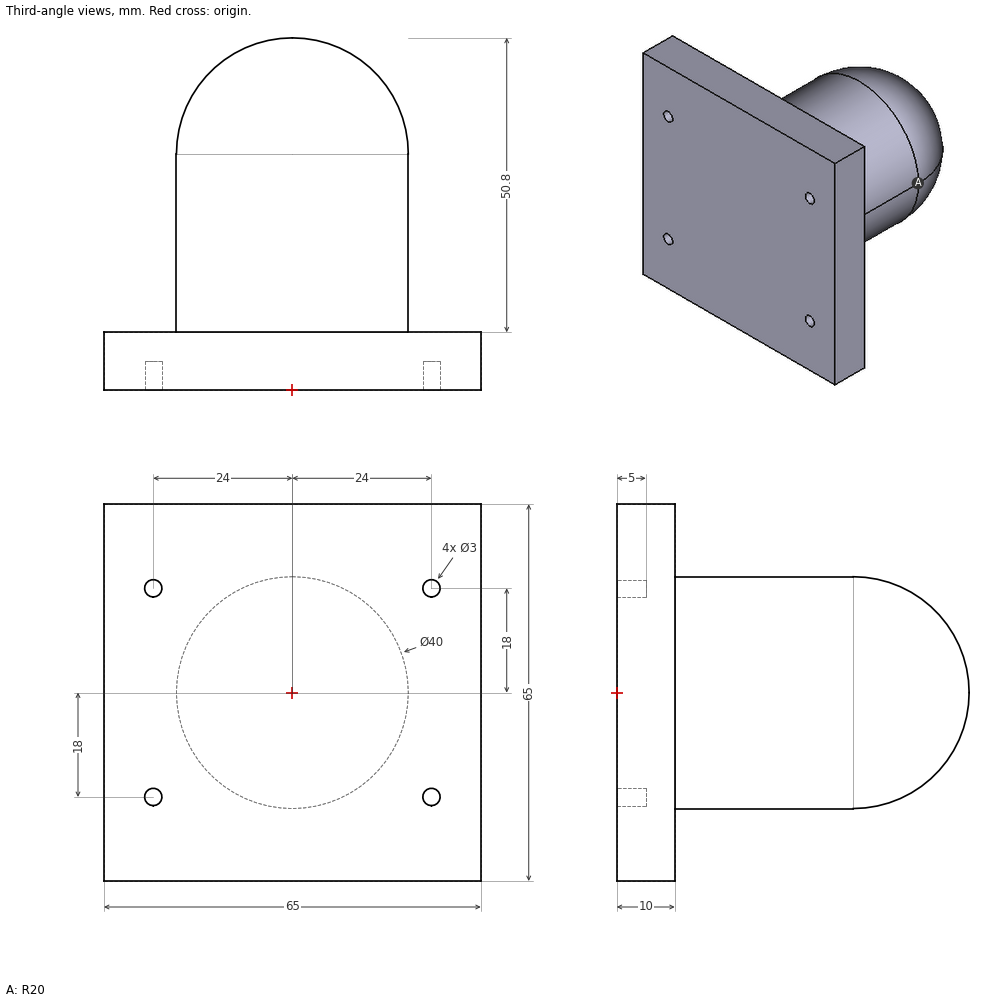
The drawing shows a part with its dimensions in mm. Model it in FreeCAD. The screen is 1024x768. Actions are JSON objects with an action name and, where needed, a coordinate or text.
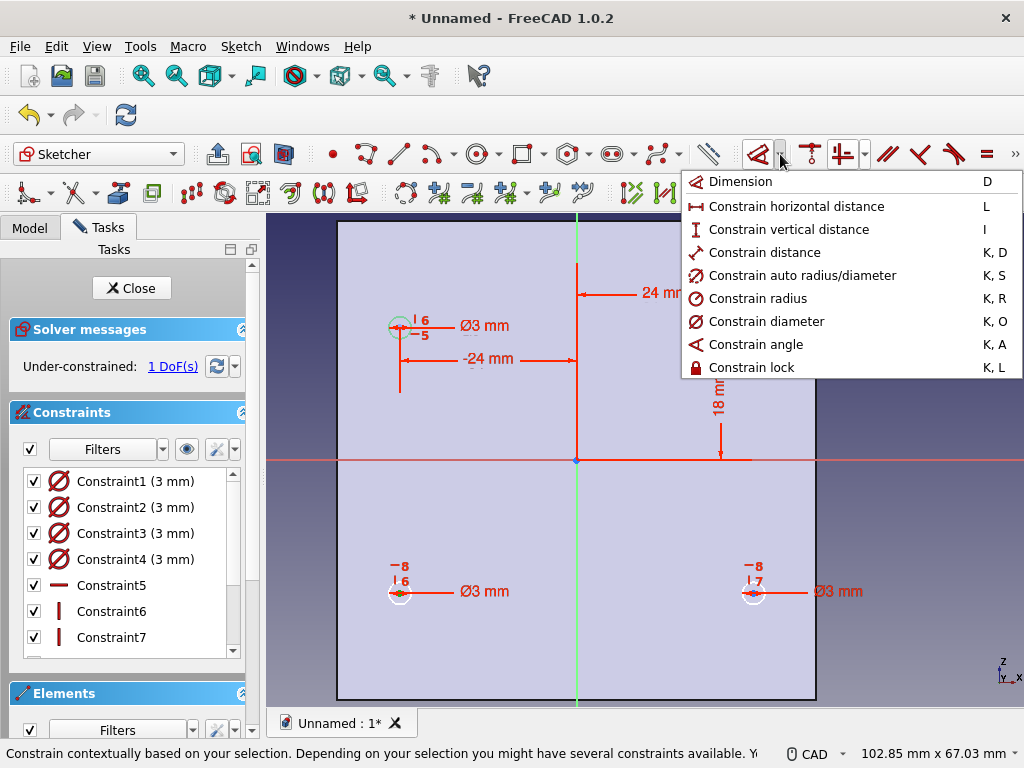
{"action": "left_click", "coordinate": [852, 230]}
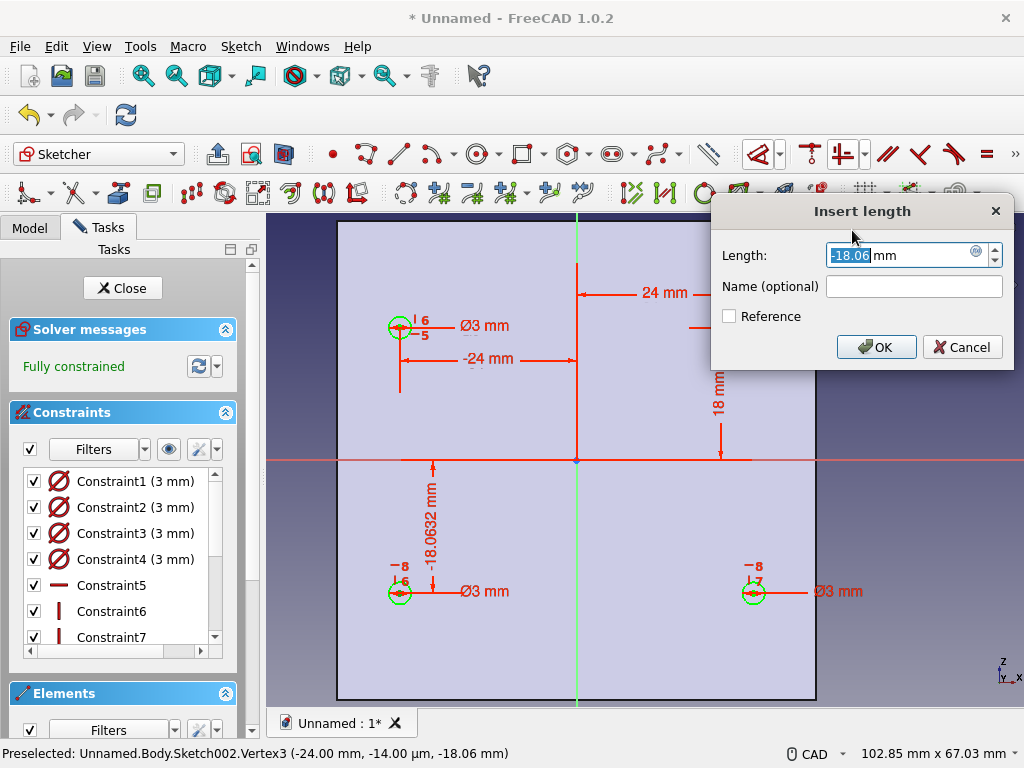
{"action": "type", "text": "-18"}
{"action": "key", "text": "Return"}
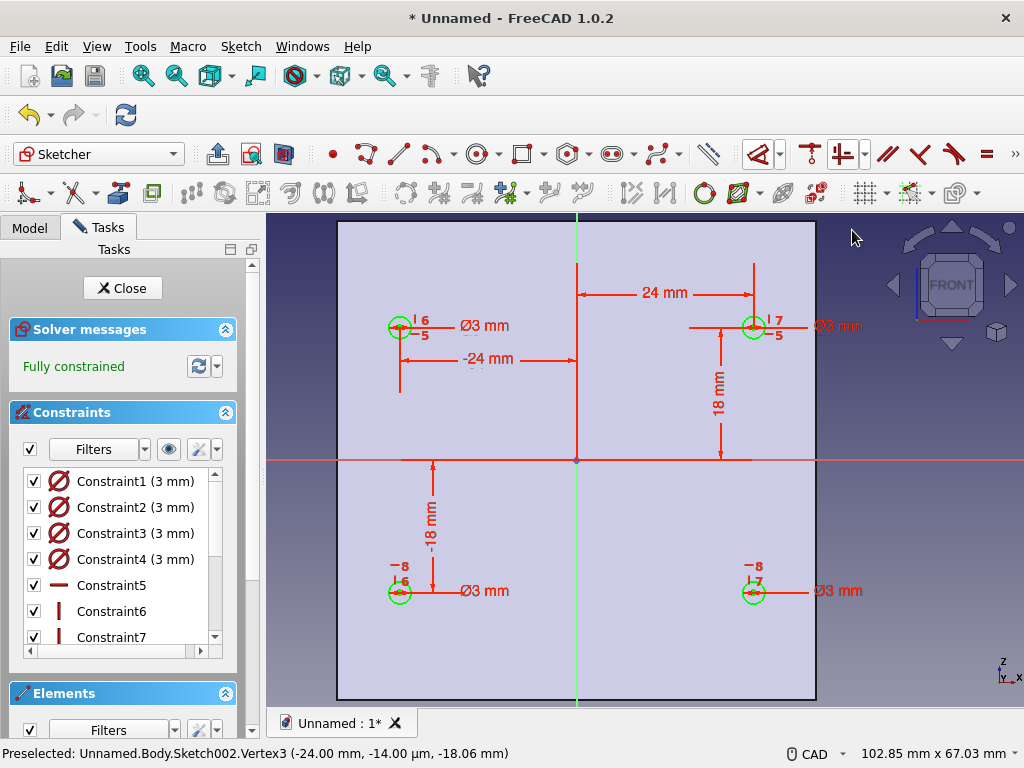
{"action": "left_click", "coordinate": [123, 288]}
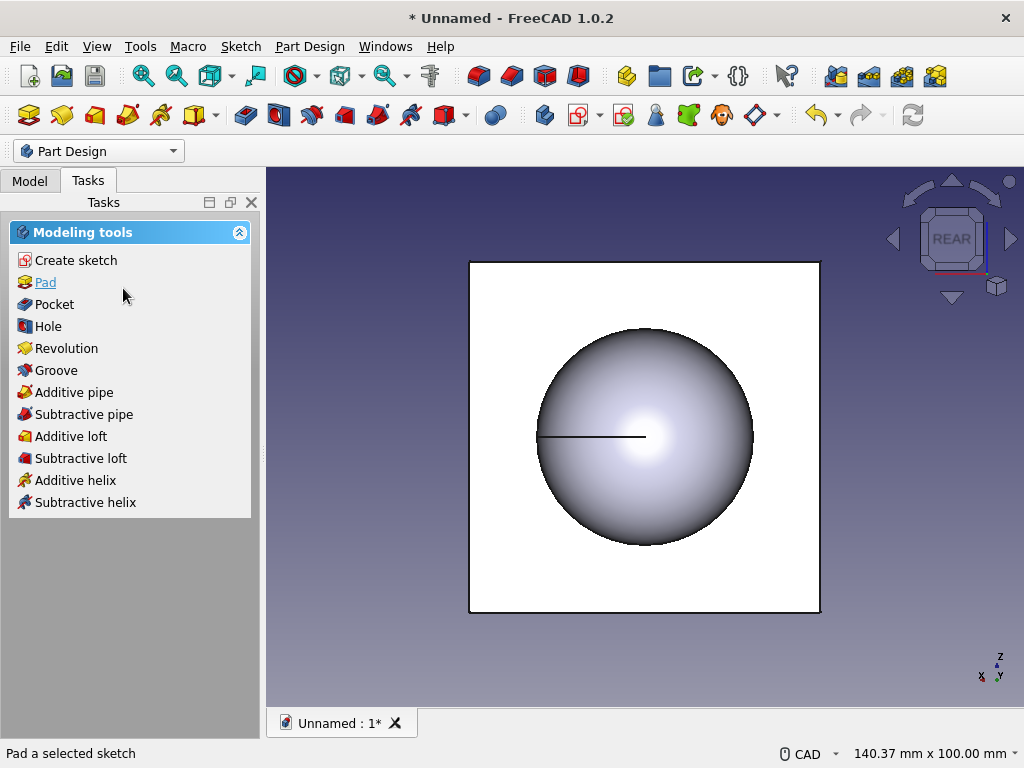
{"action": "left_click", "coordinate": [246, 116]}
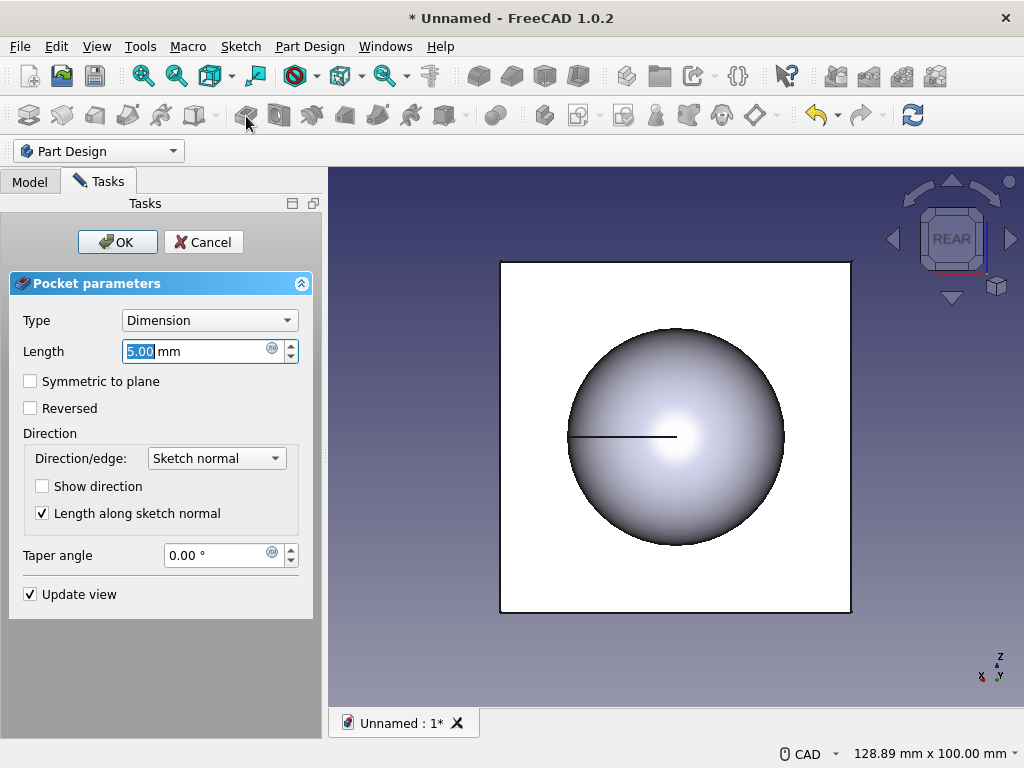
{"action": "type", "text": "5"}
{"action": "key", "text": "Tab"}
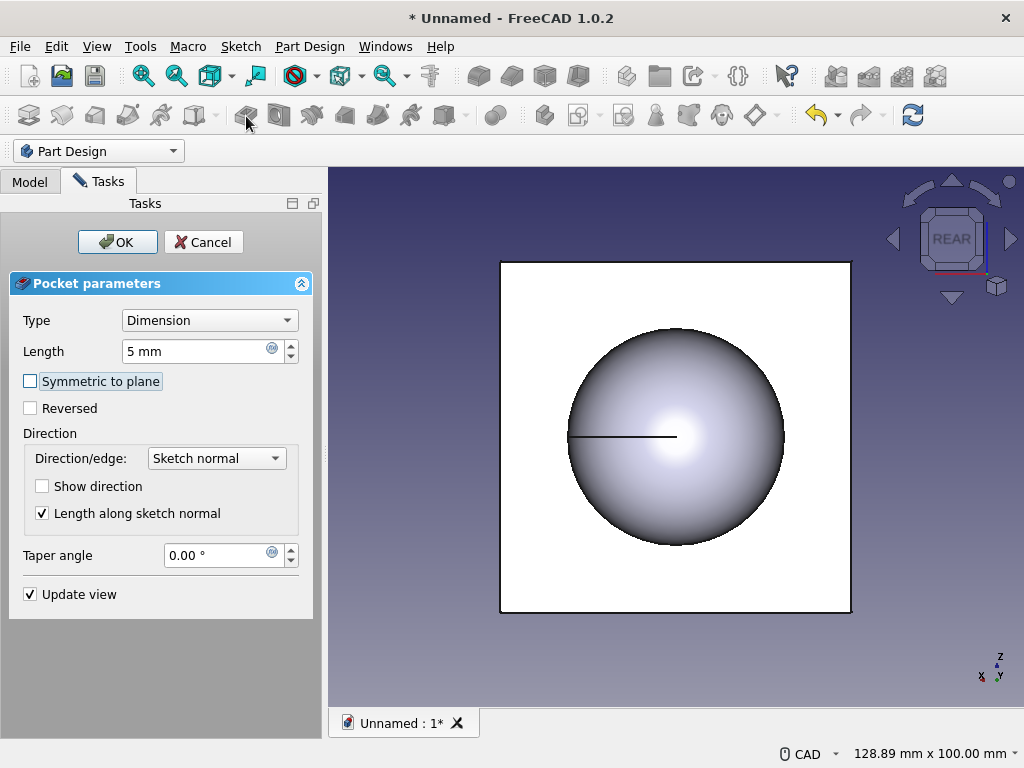
{"action": "left_click", "coordinate": [118, 242]}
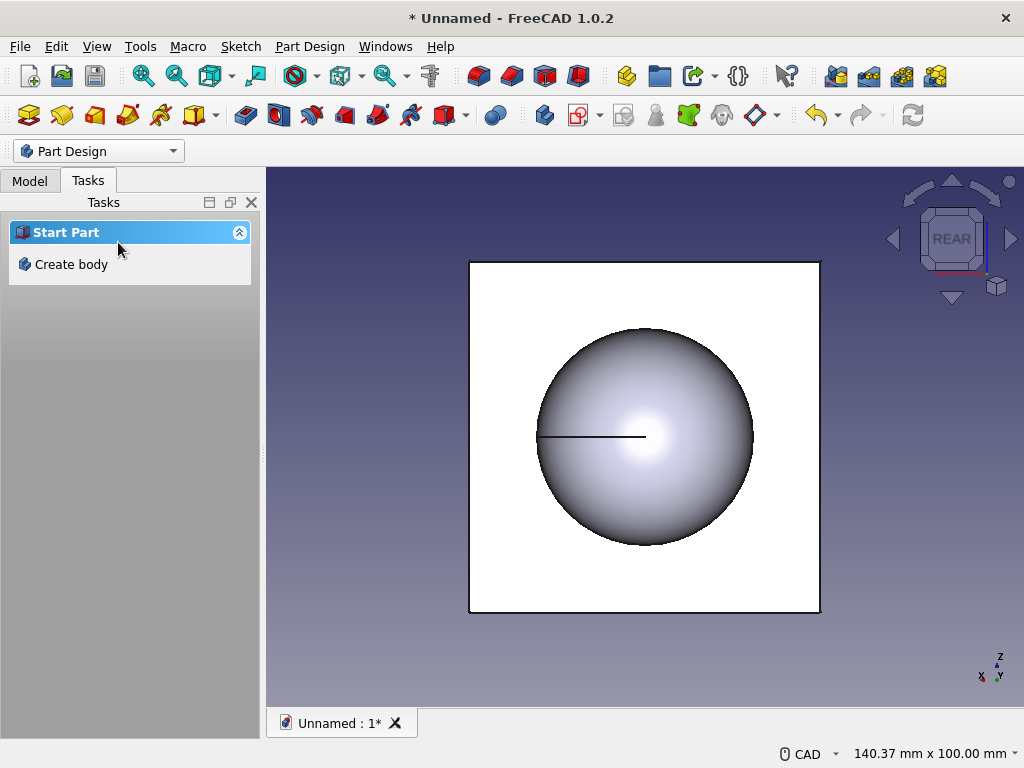
{"action": "key", "text": "0"}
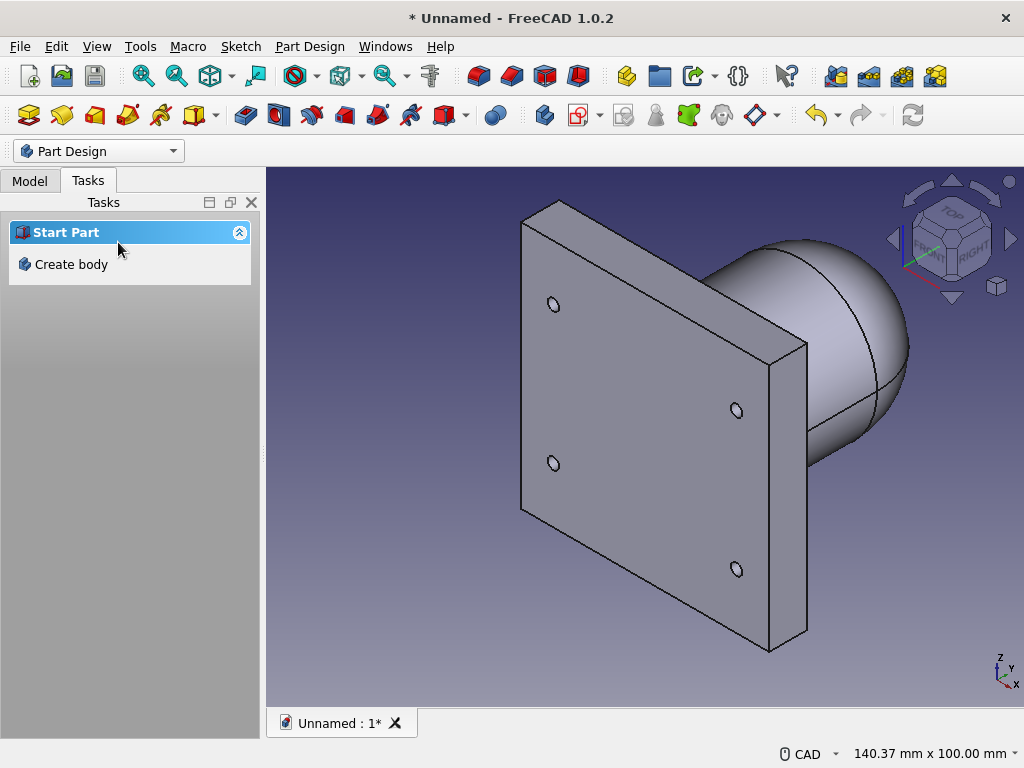
{"action": "left_click", "coordinate": [144, 76]}